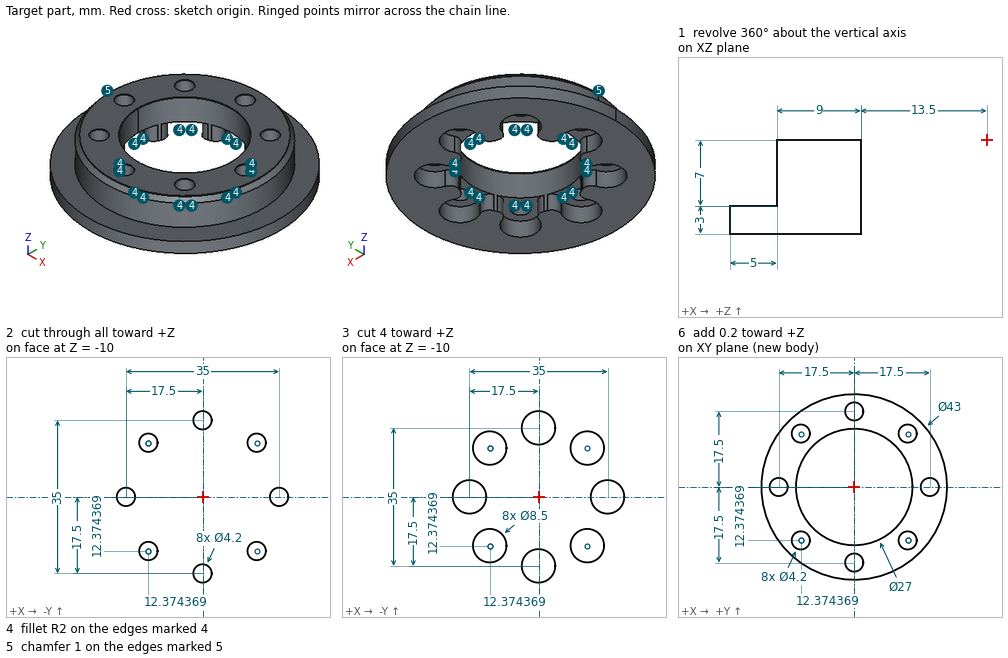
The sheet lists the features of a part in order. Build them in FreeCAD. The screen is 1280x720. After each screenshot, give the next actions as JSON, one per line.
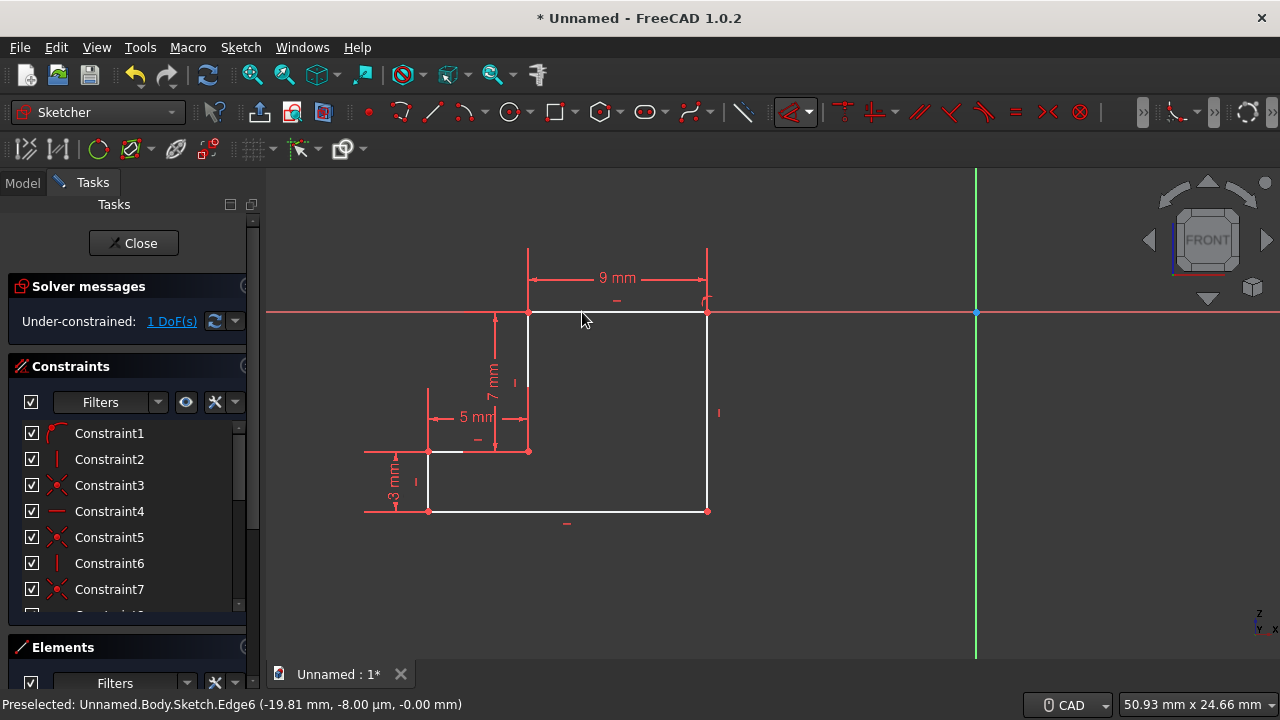
{"action": "left_click", "coordinate": [707, 312]}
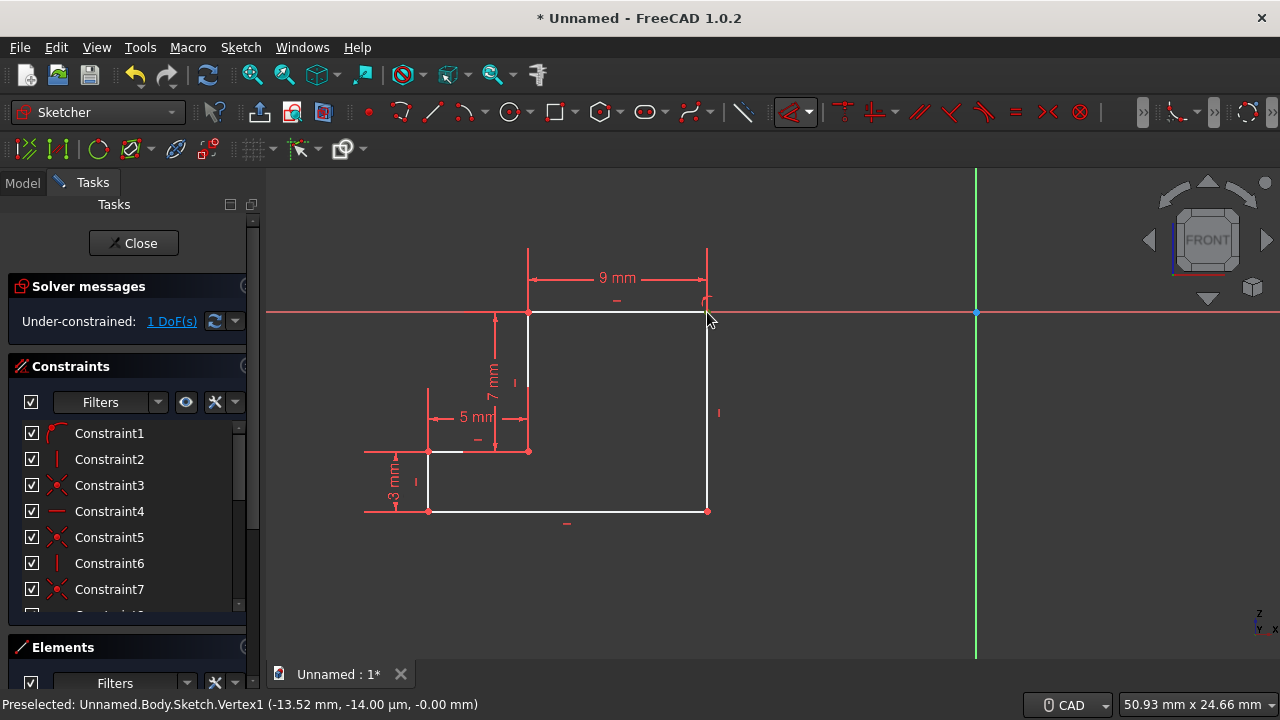
{"action": "key", "text": "l"}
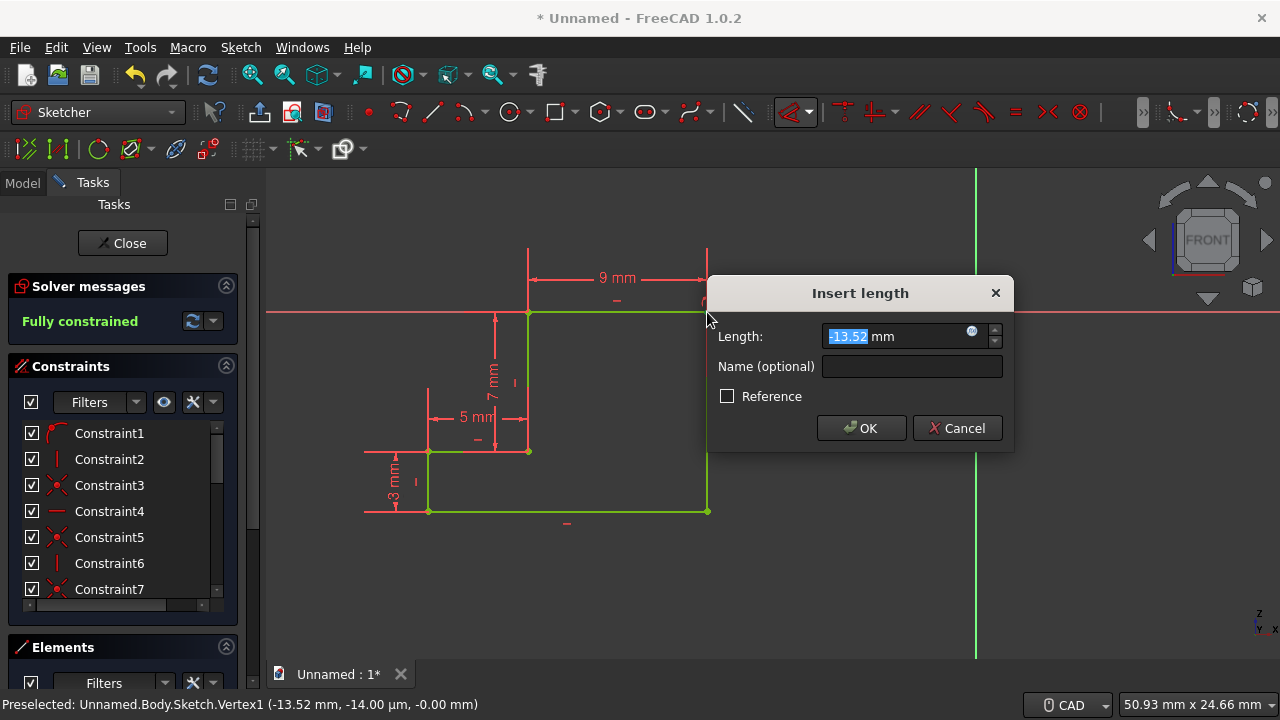
{"action": "type", "text": "-13.5"}
{"action": "key", "text": "Return"}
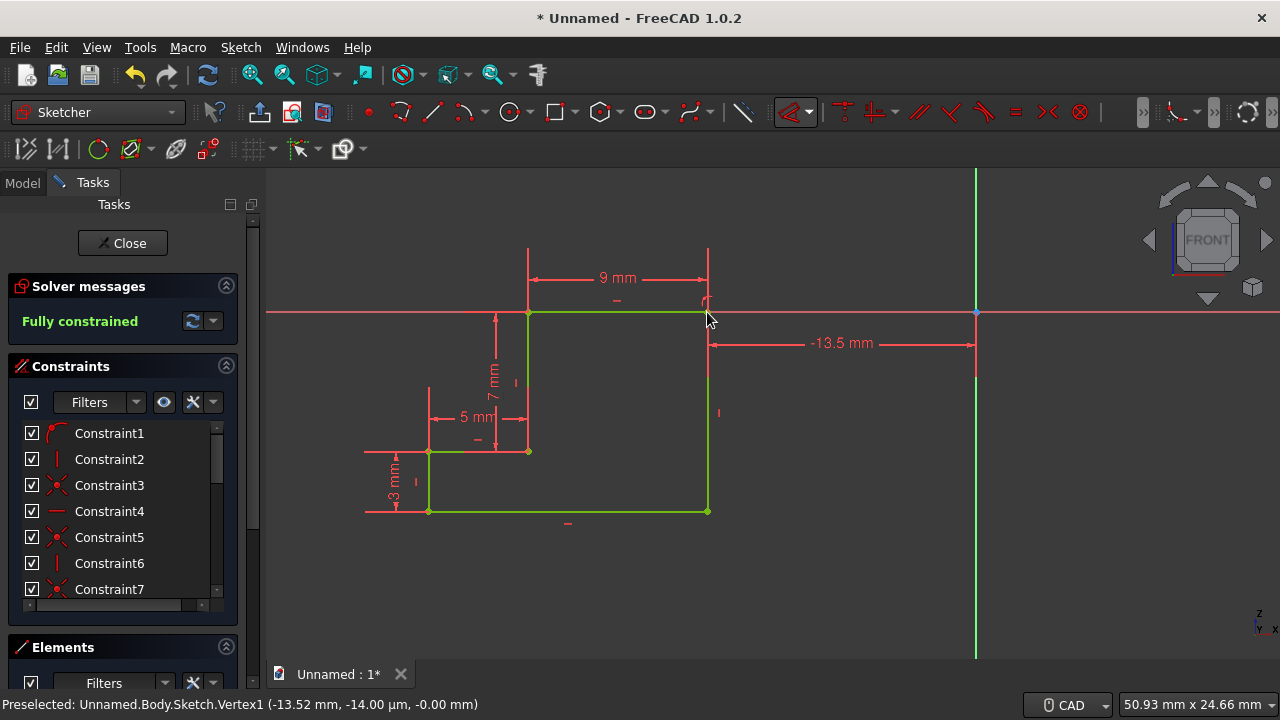
{"action": "left_click", "coordinate": [123, 243]}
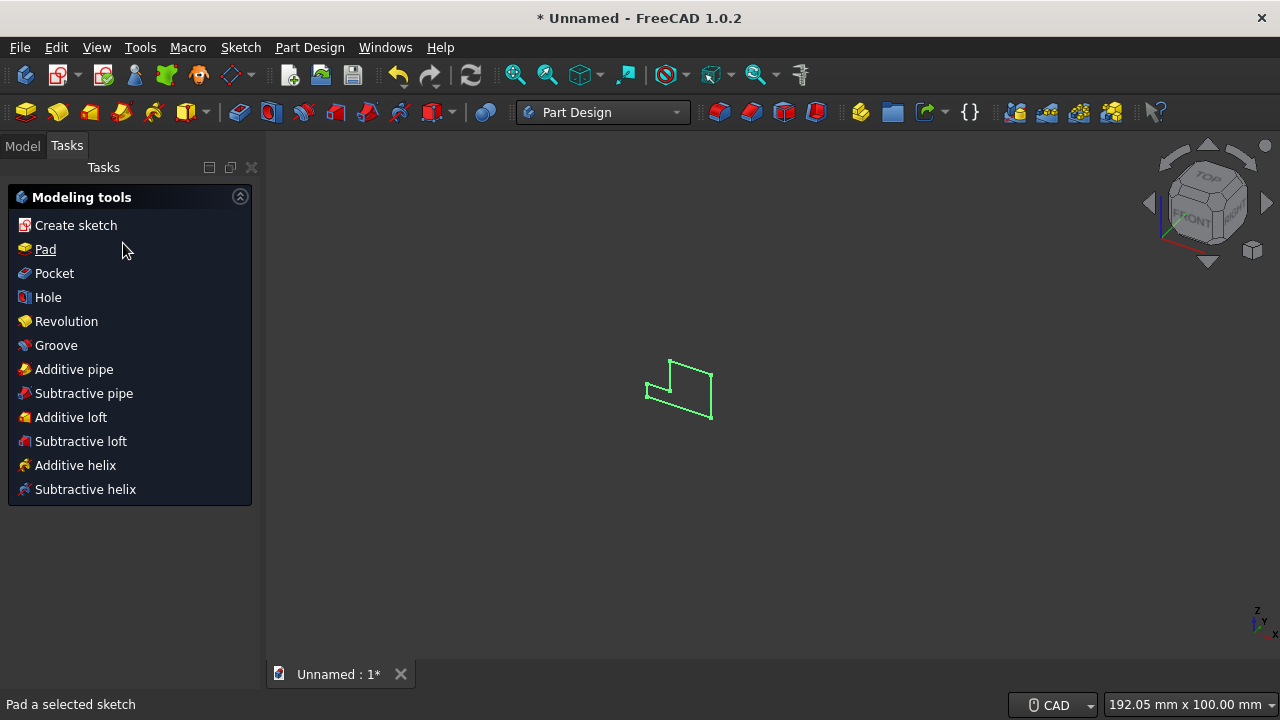
{"action": "left_click", "coordinate": [58, 112]}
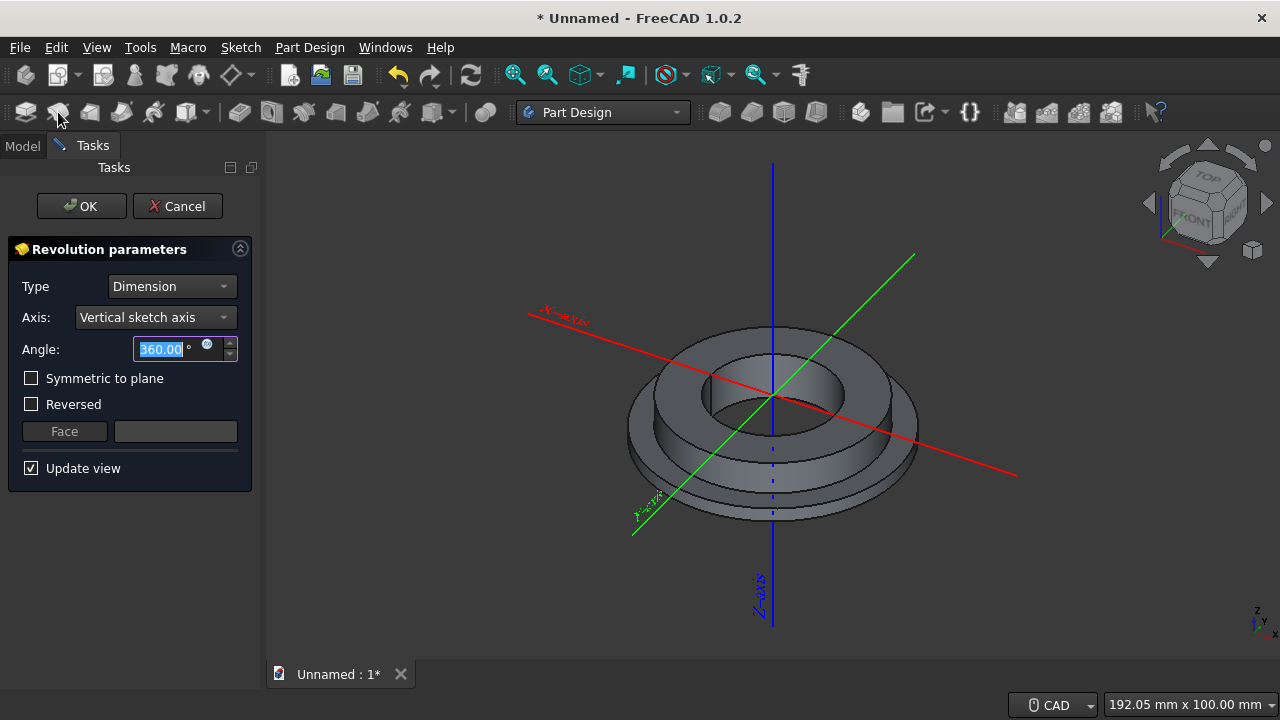
{"action": "left_click", "coordinate": [82, 206]}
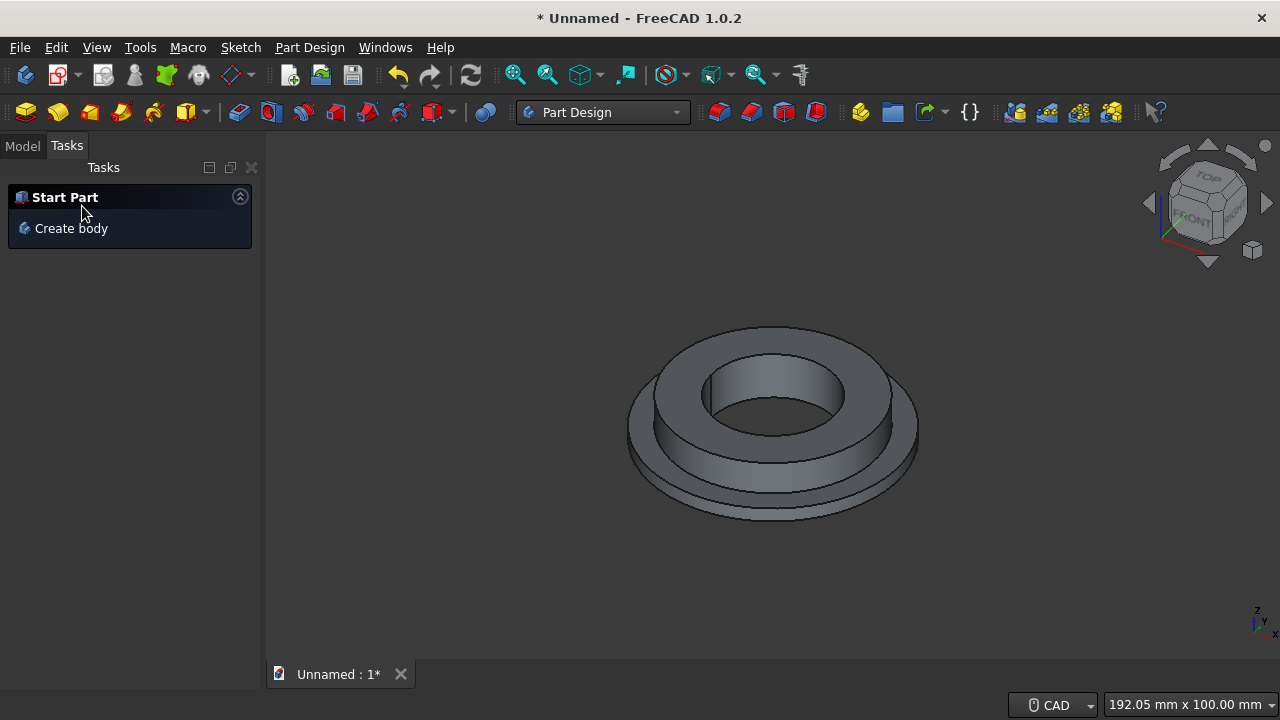
{"action": "key", "text": "5"}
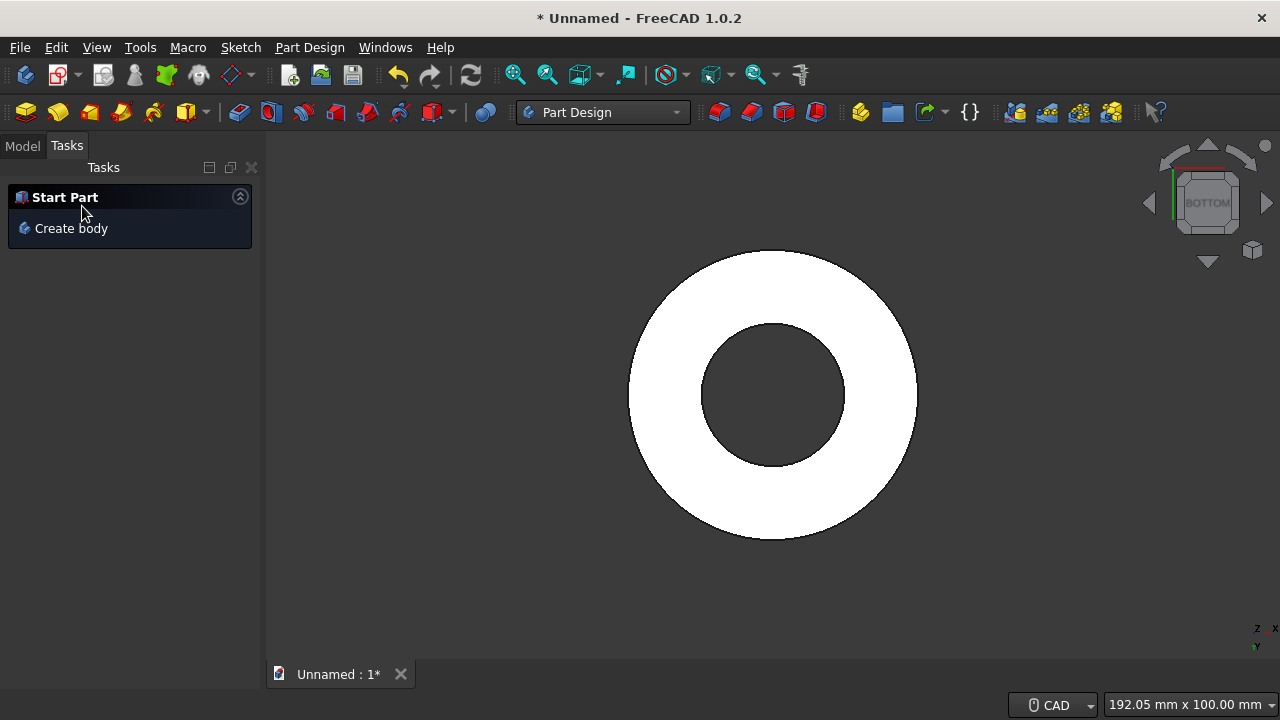
{"action": "left_click", "coordinate": [690, 311]}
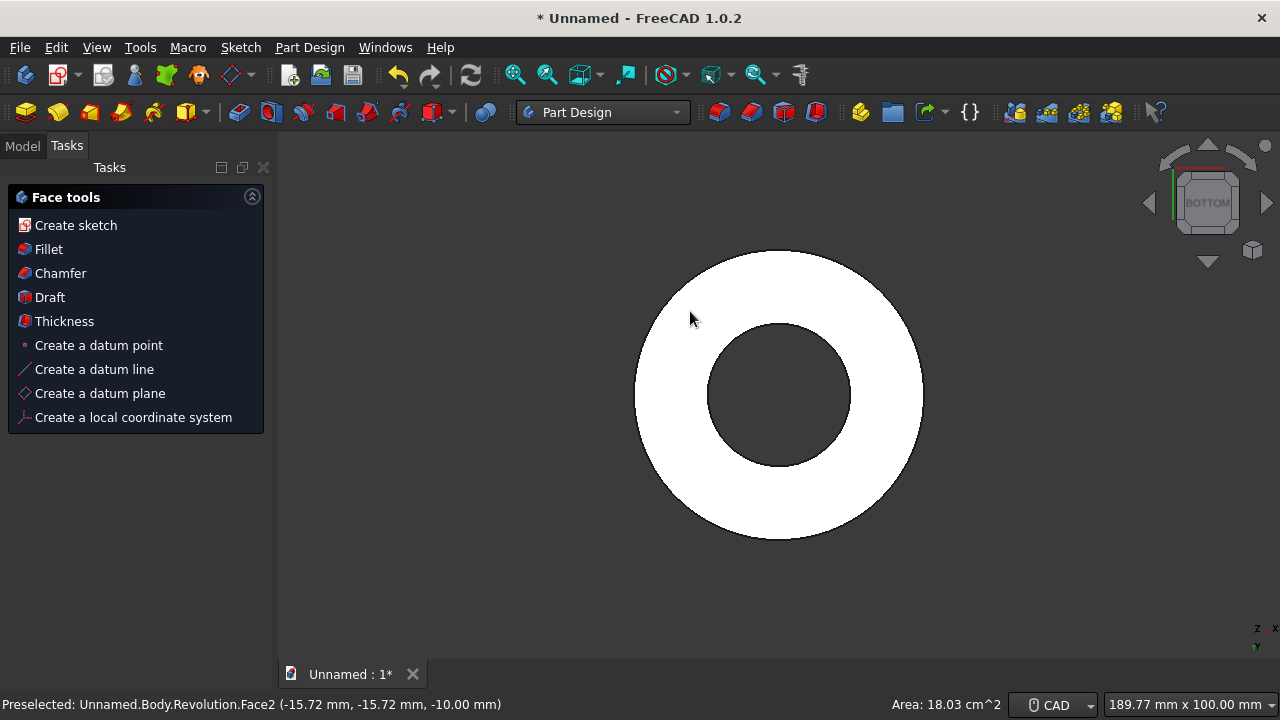
{"action": "left_click", "coordinate": [58, 76]}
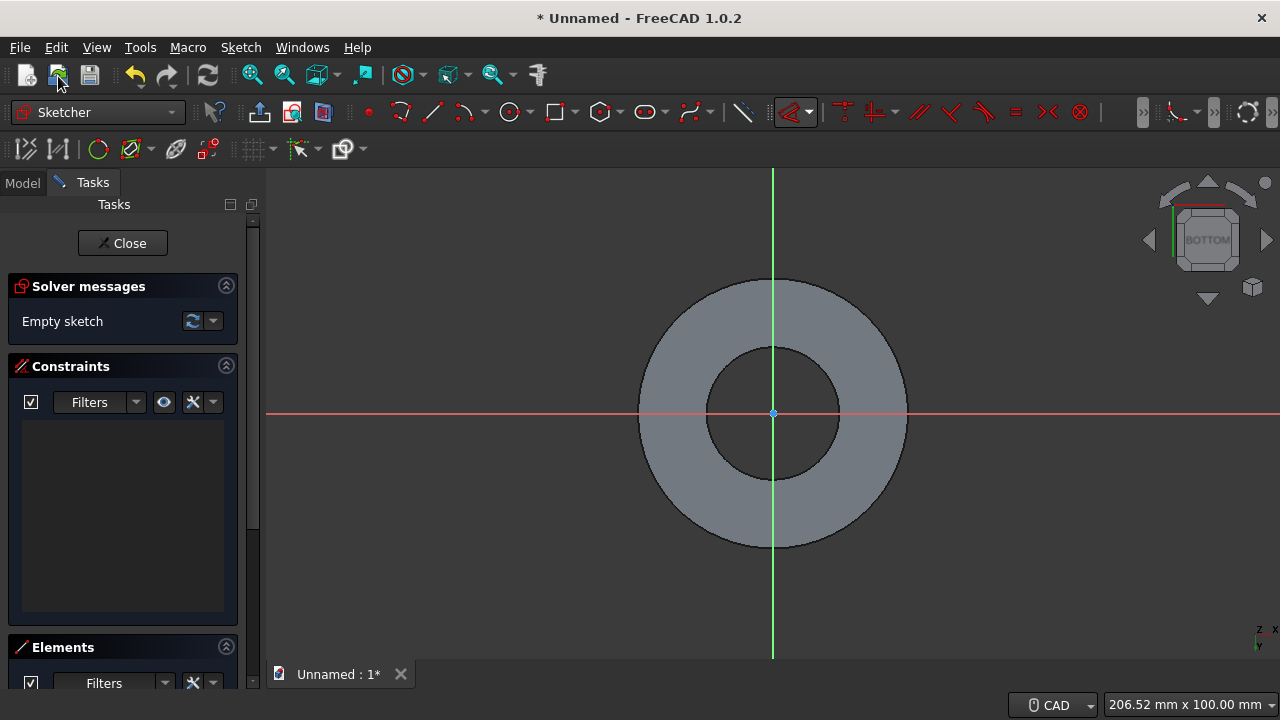
{"action": "scroll", "coordinate": [912, 413], "scroll_direction": "up", "scroll_amount": 2}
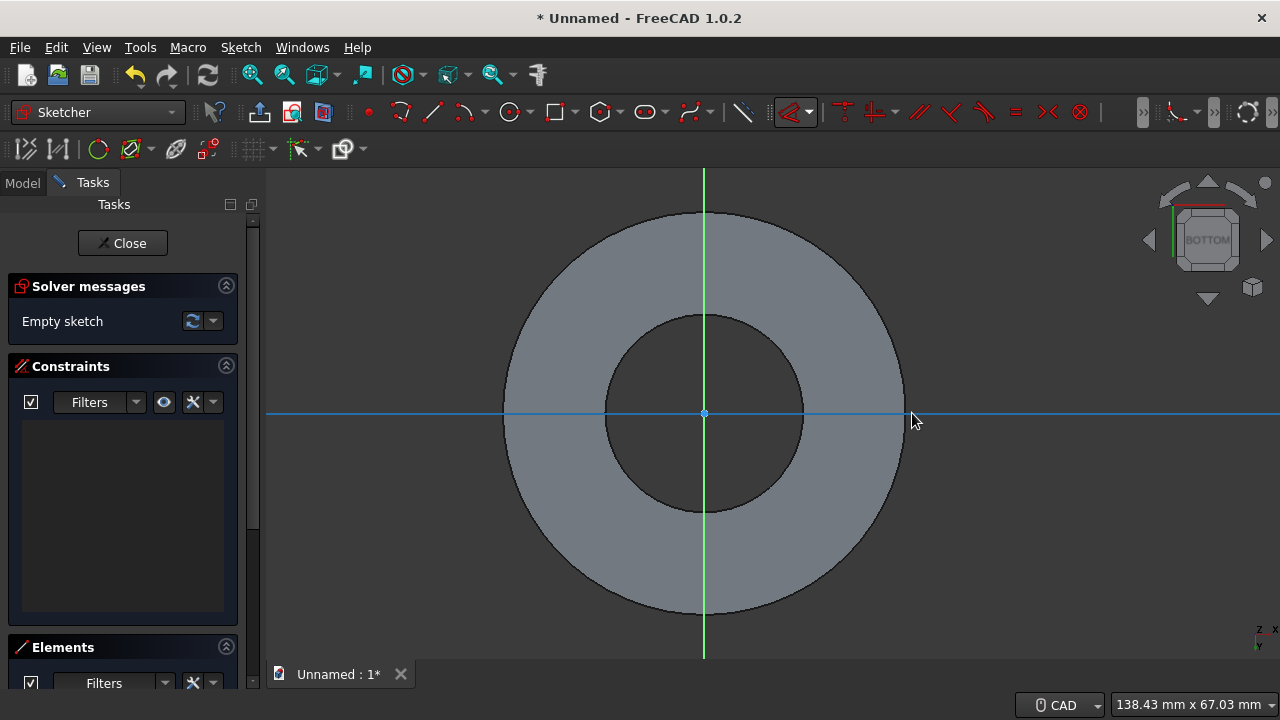
{"action": "key", "text": "g c"}